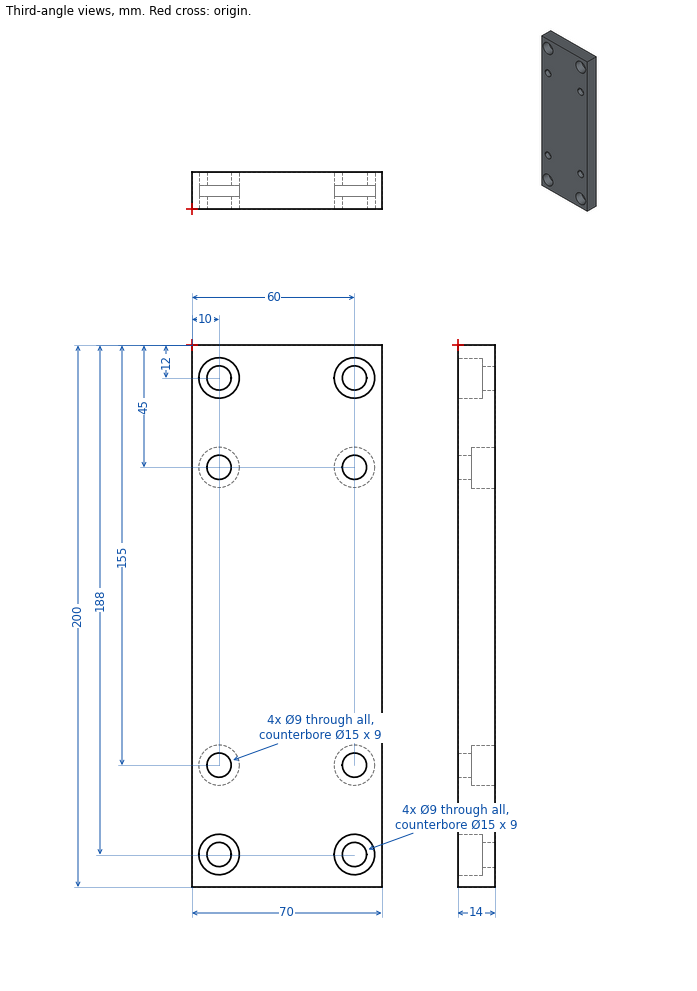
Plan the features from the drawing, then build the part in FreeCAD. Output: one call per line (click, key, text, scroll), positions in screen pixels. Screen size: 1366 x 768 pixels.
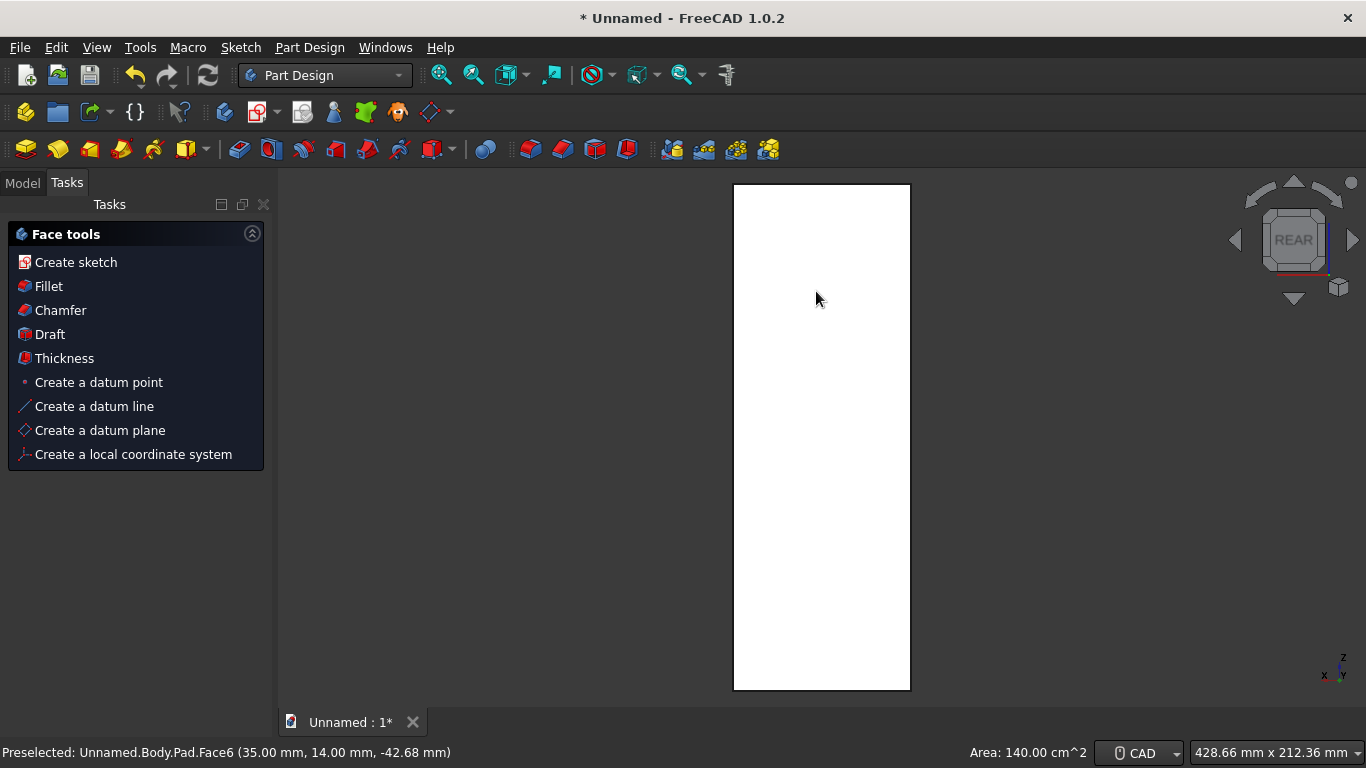
click(258, 112)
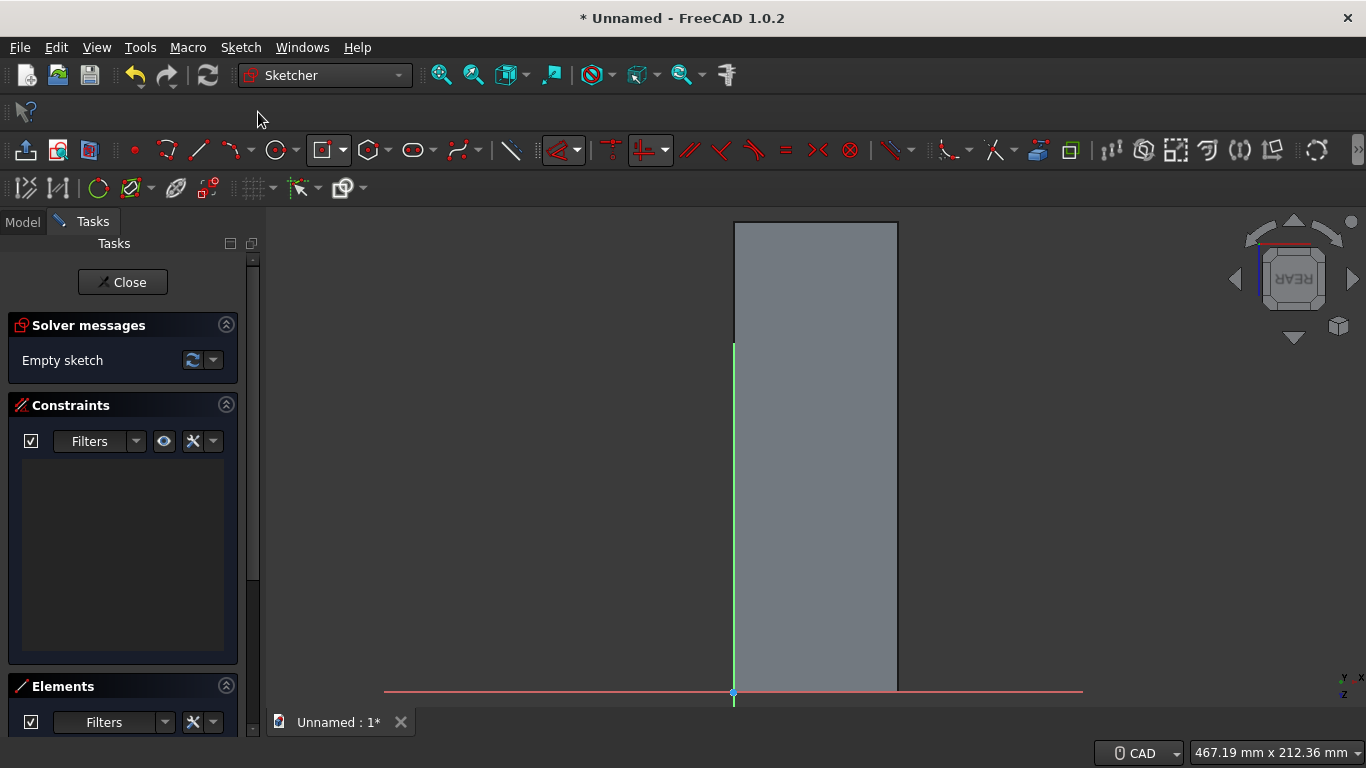
scroll(467, 242, down, 1)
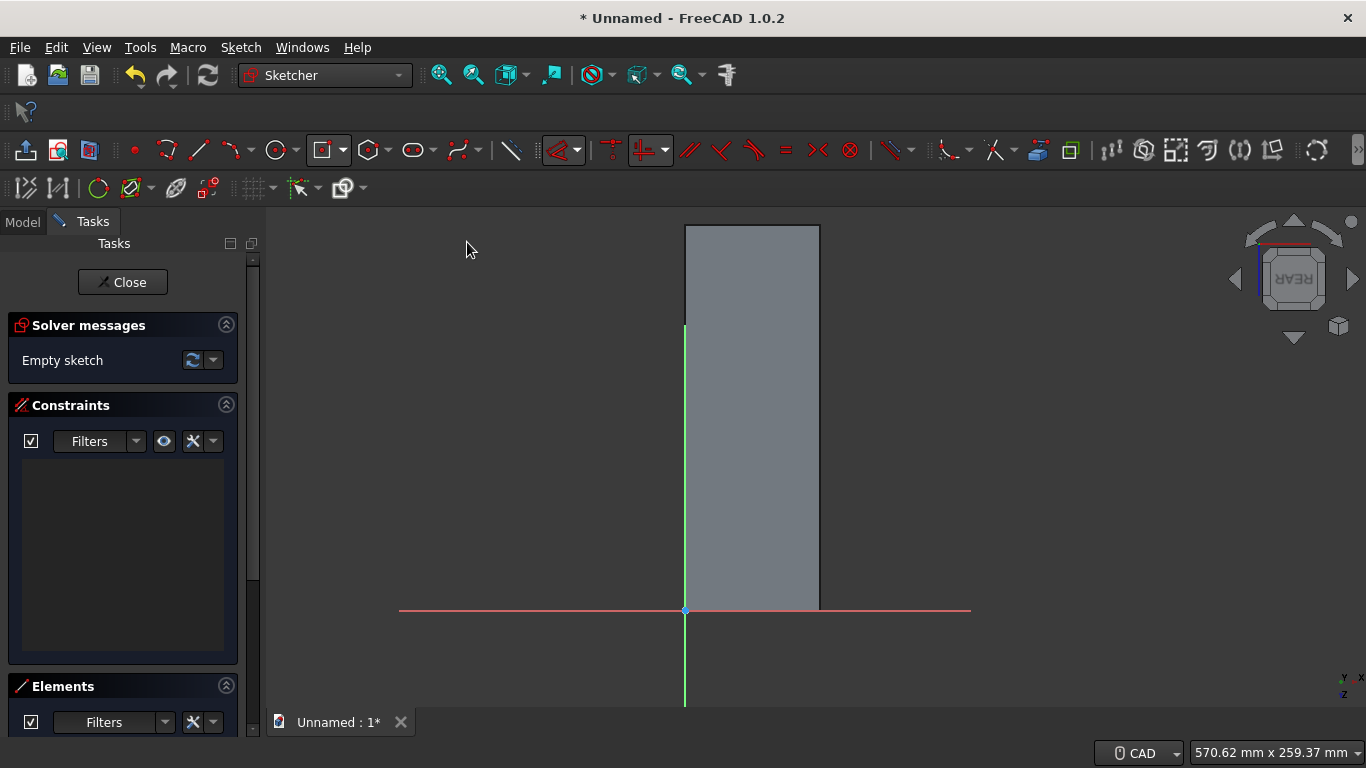
key(g)
key(c)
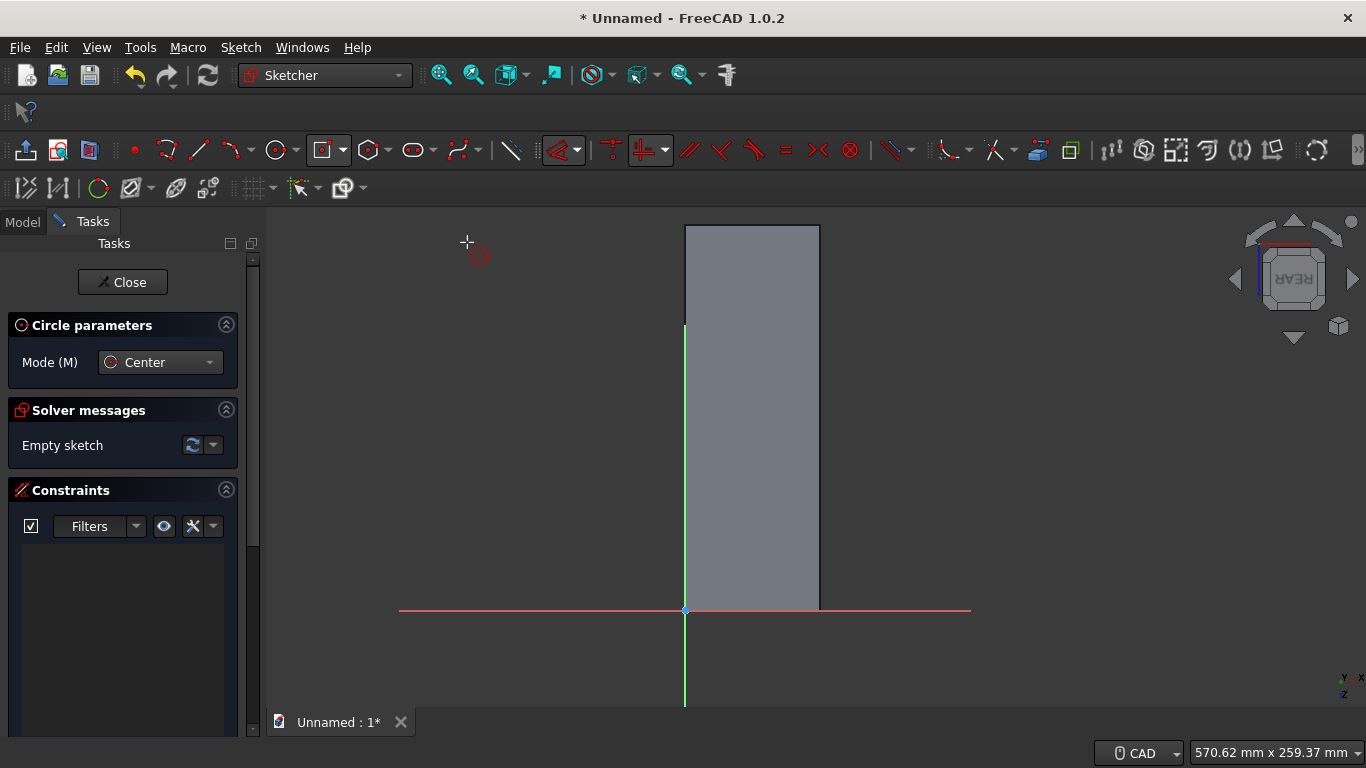
scroll(705, 312, up, 5)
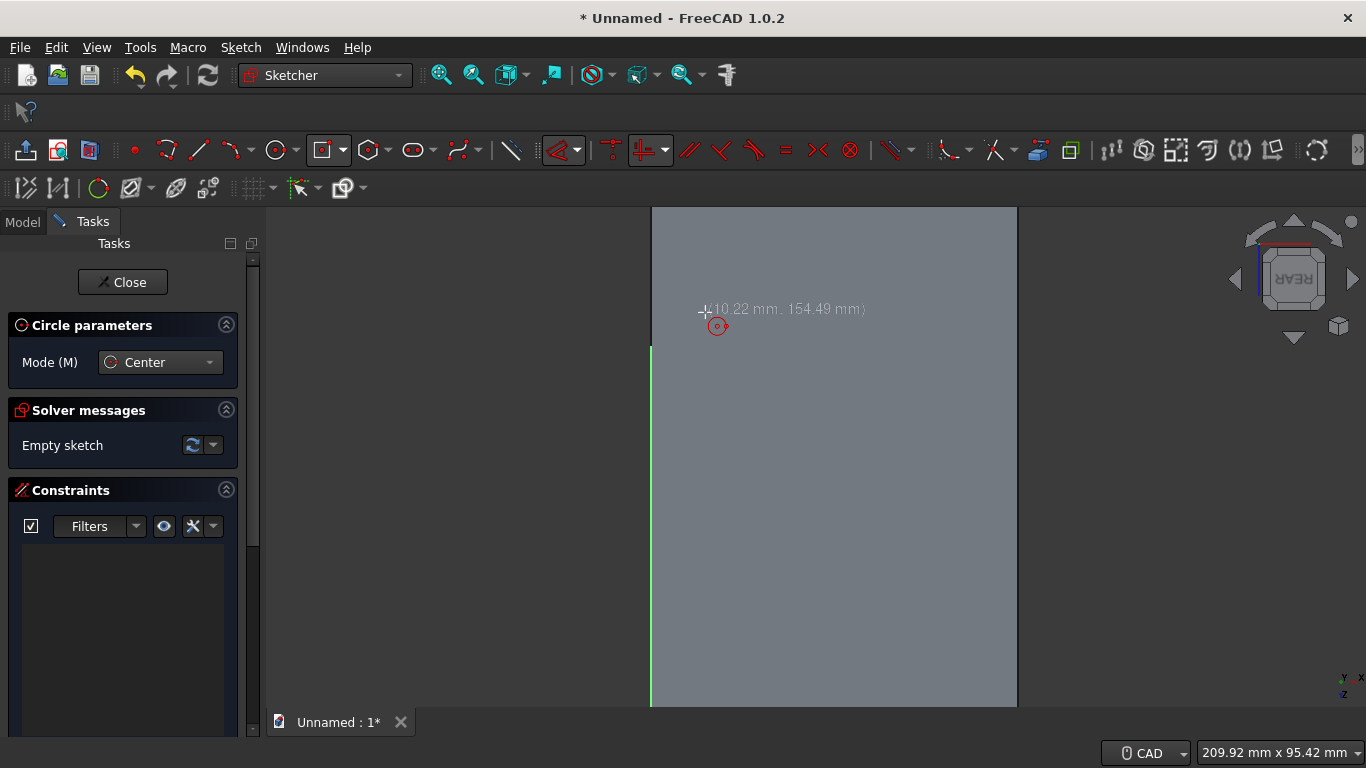
click(703, 312)
click(720, 295)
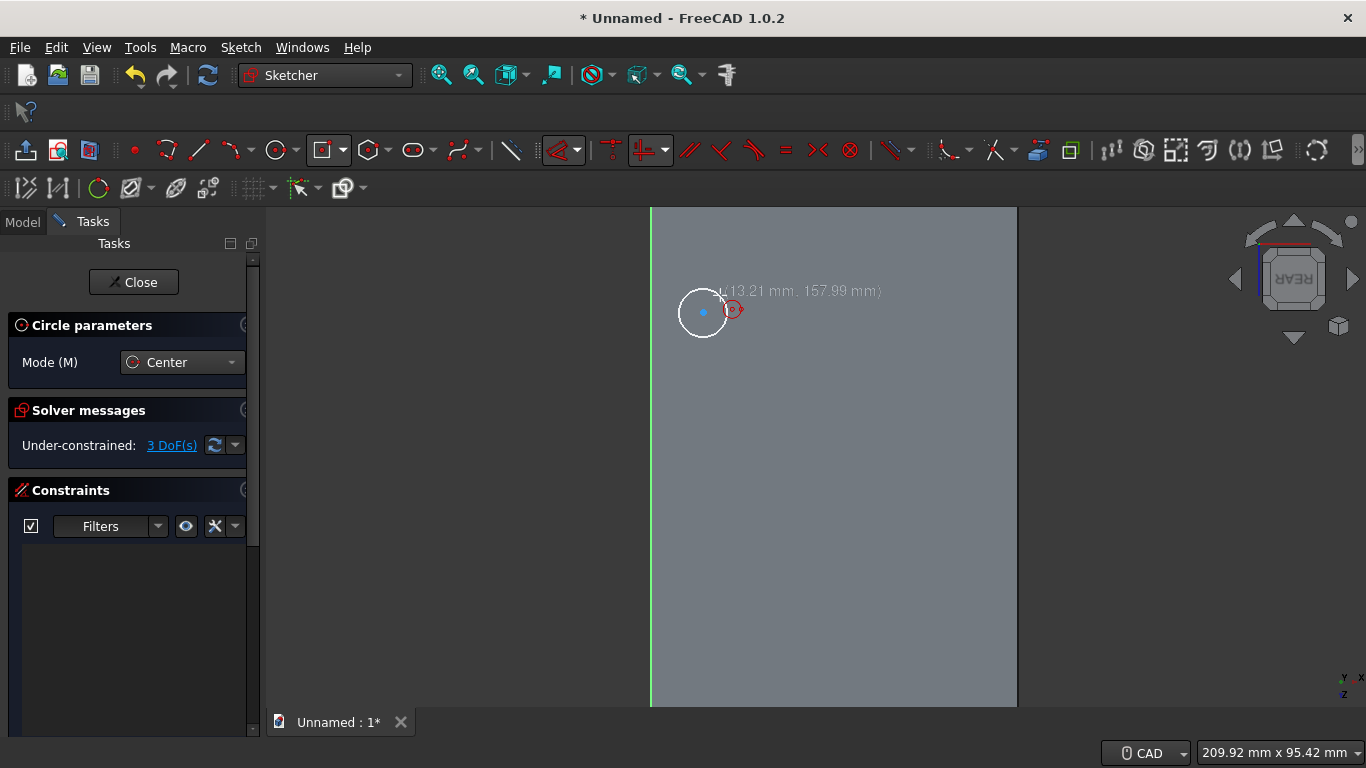
click(965, 312)
click(982, 295)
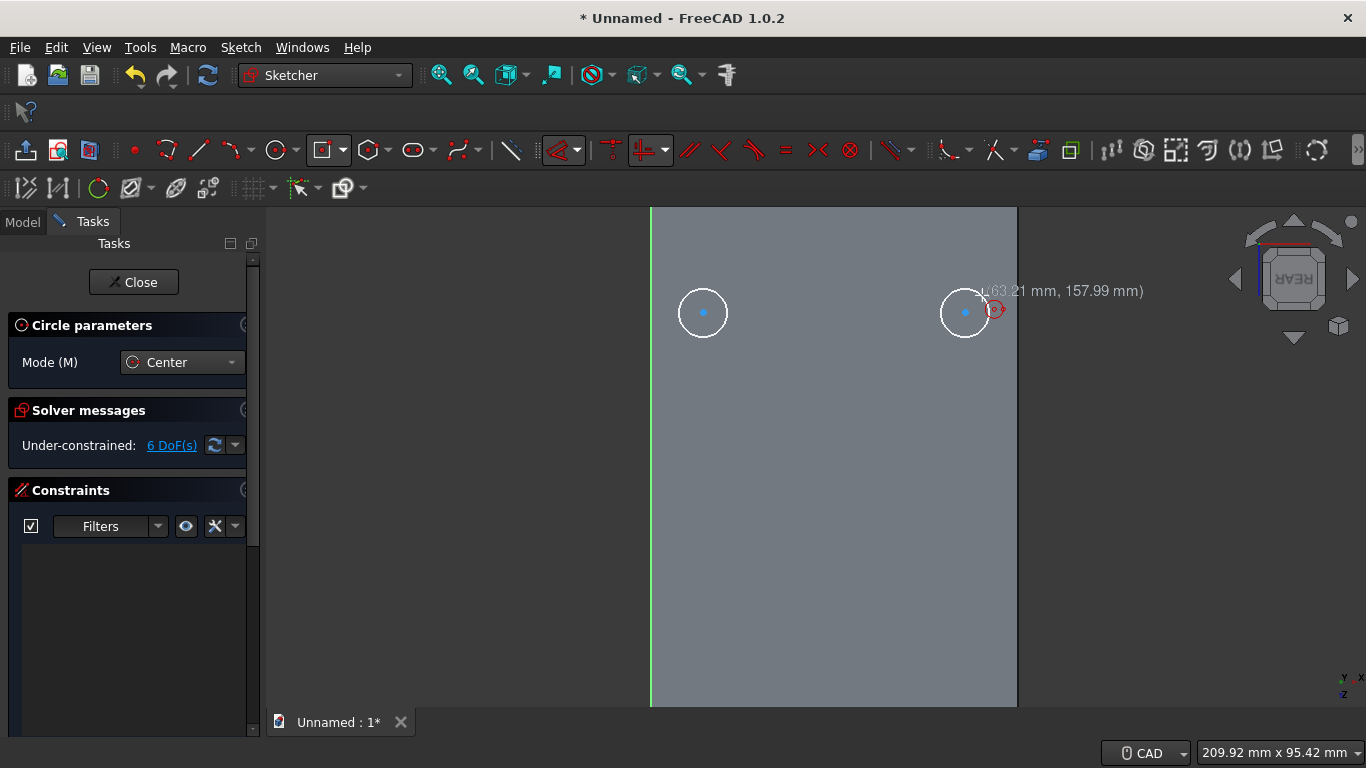
scroll(705, 312, down, 5)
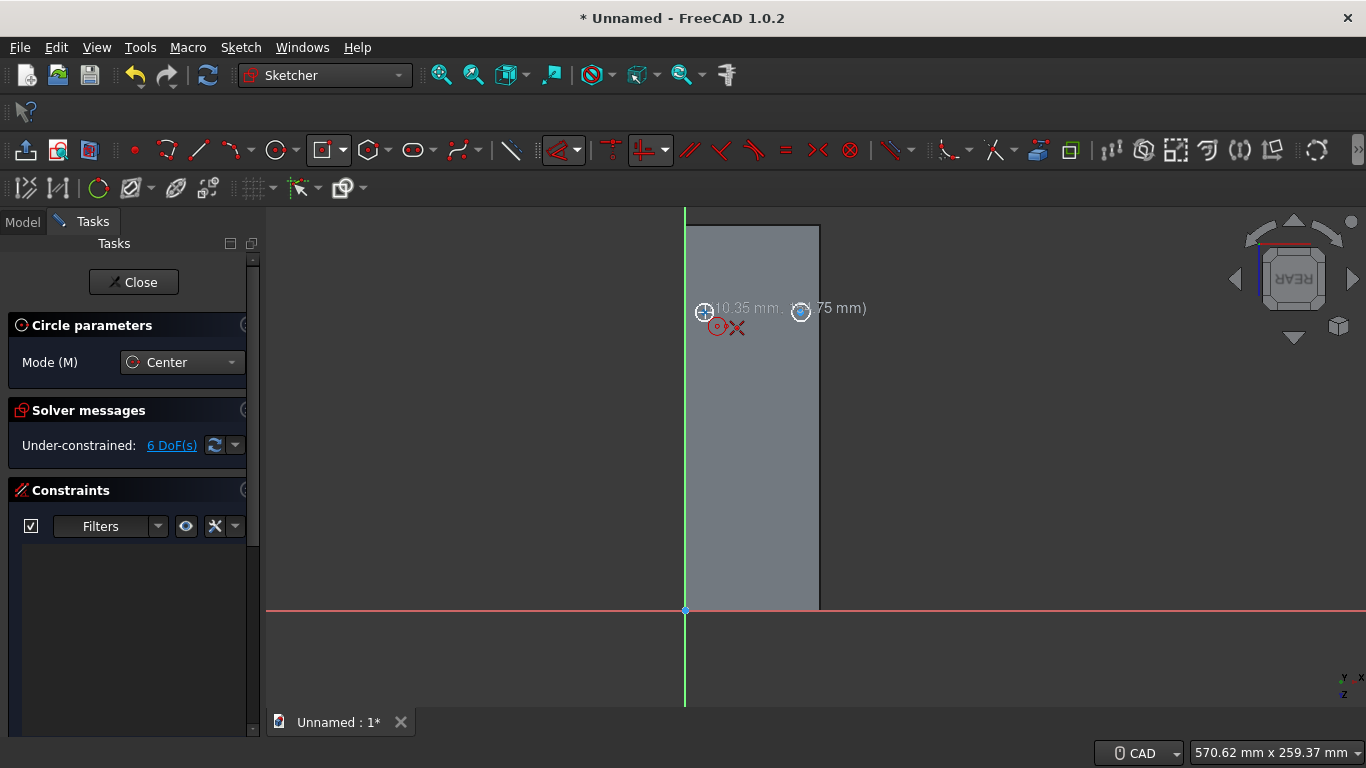
scroll(801, 524, up, 5)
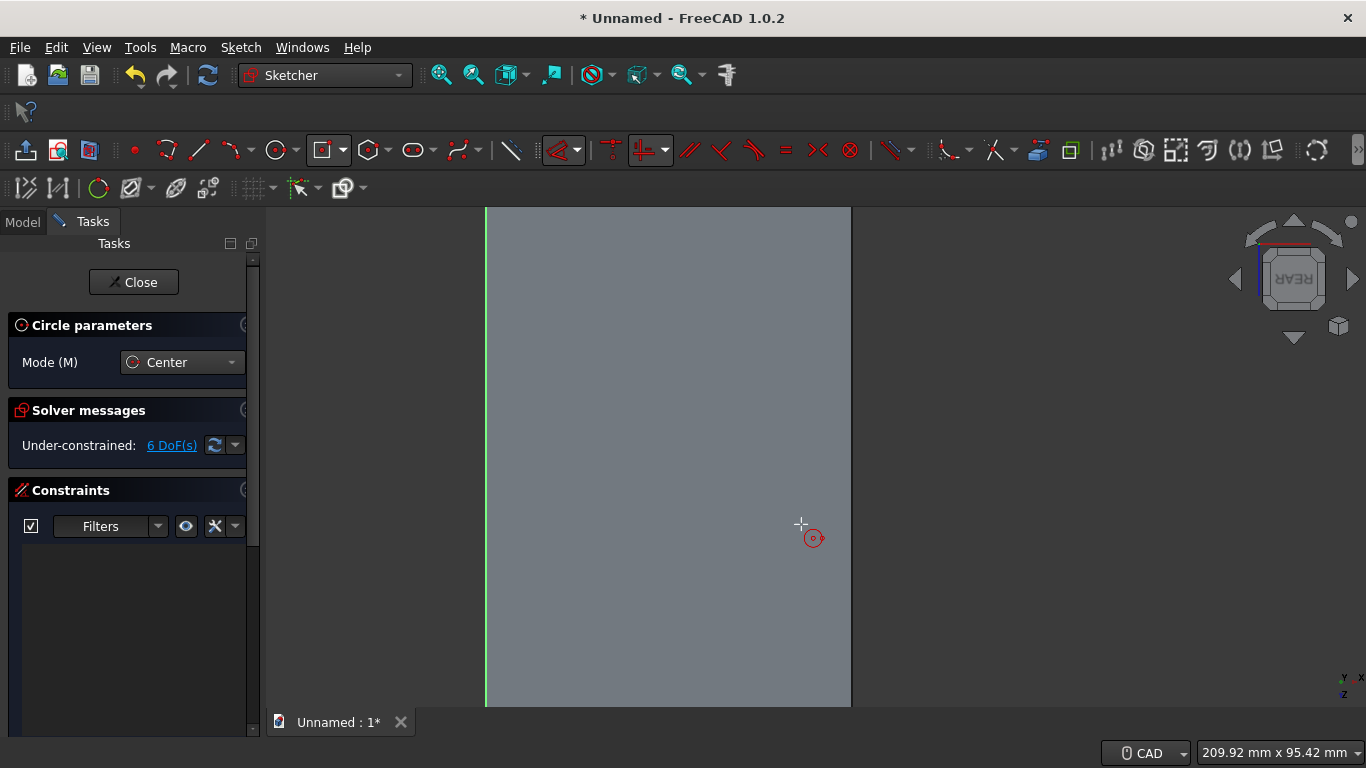
click(800, 523)
click(817, 506)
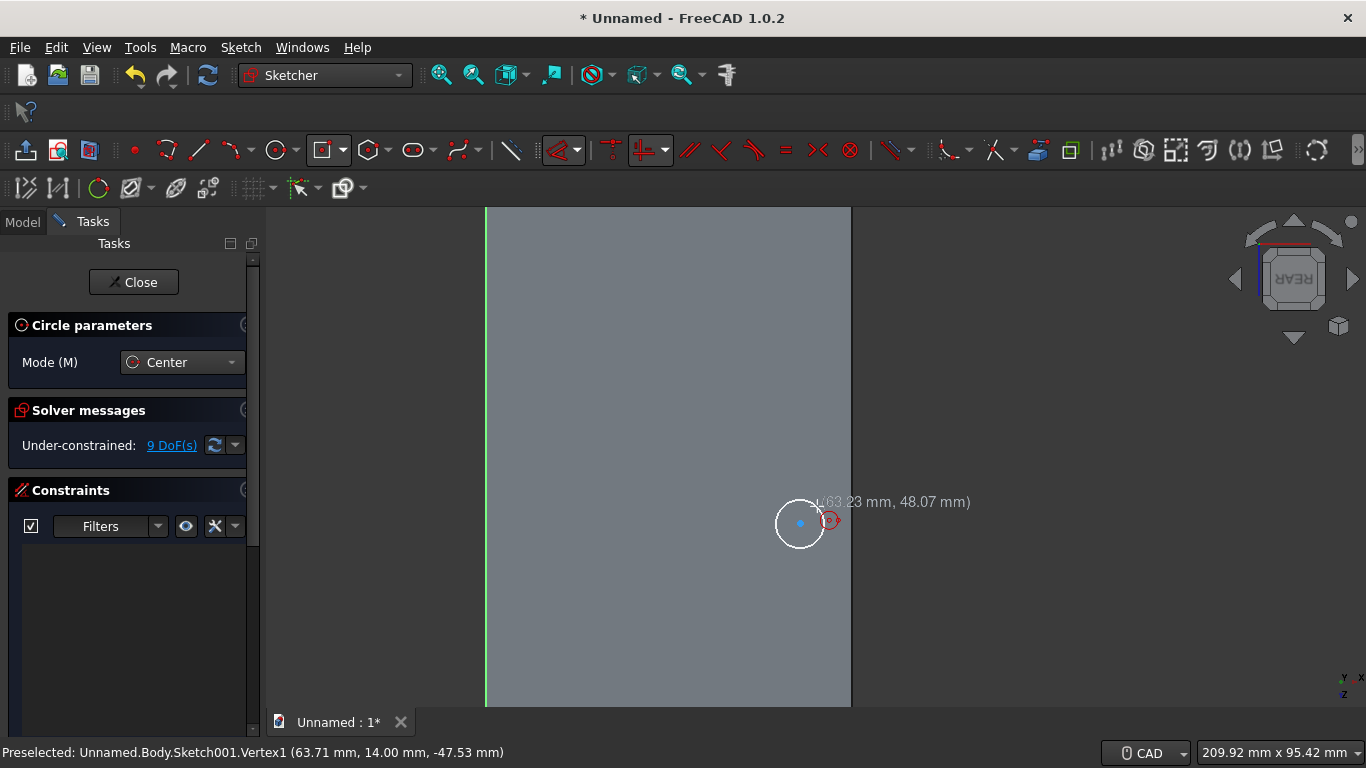
click(538, 523)
click(555, 506)
key(Escape)